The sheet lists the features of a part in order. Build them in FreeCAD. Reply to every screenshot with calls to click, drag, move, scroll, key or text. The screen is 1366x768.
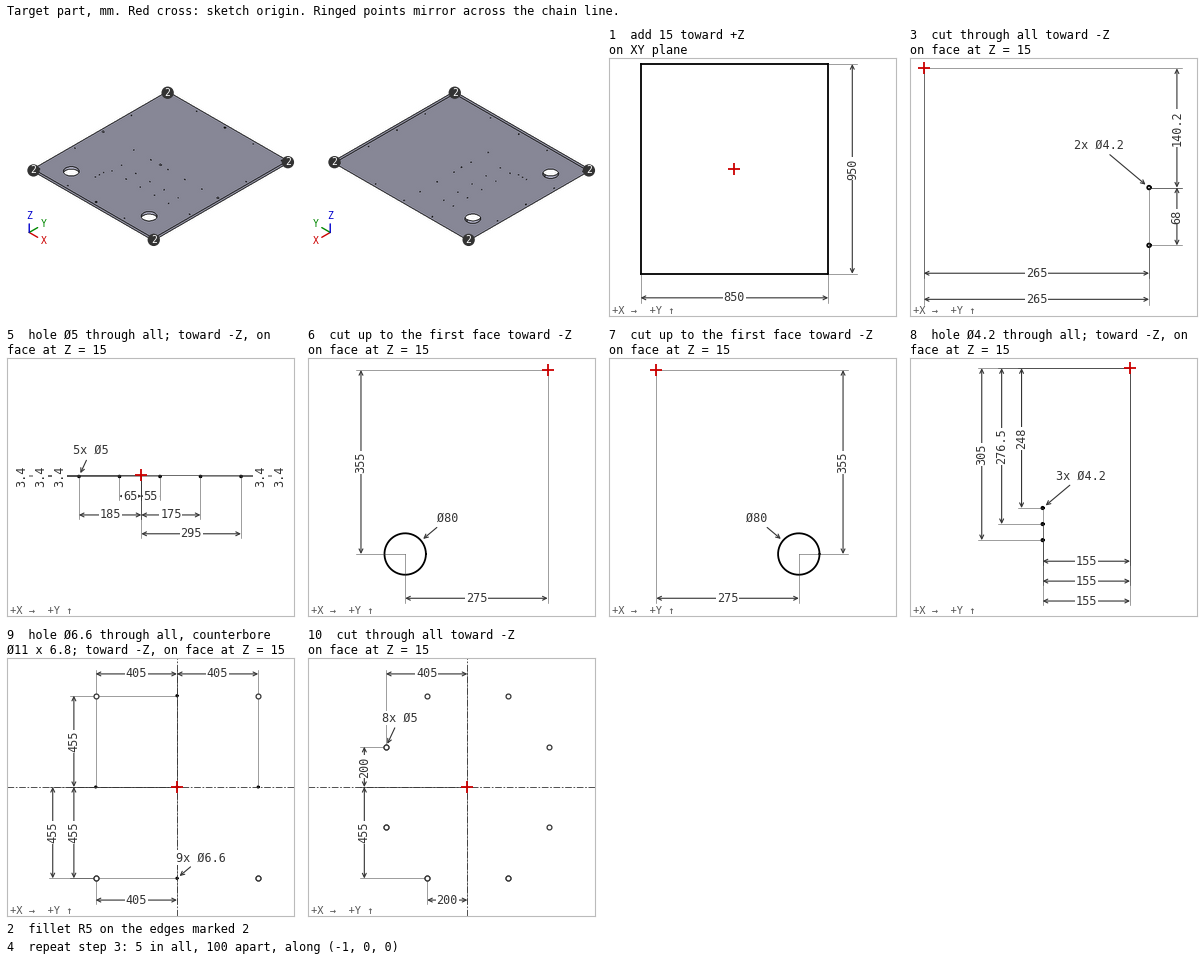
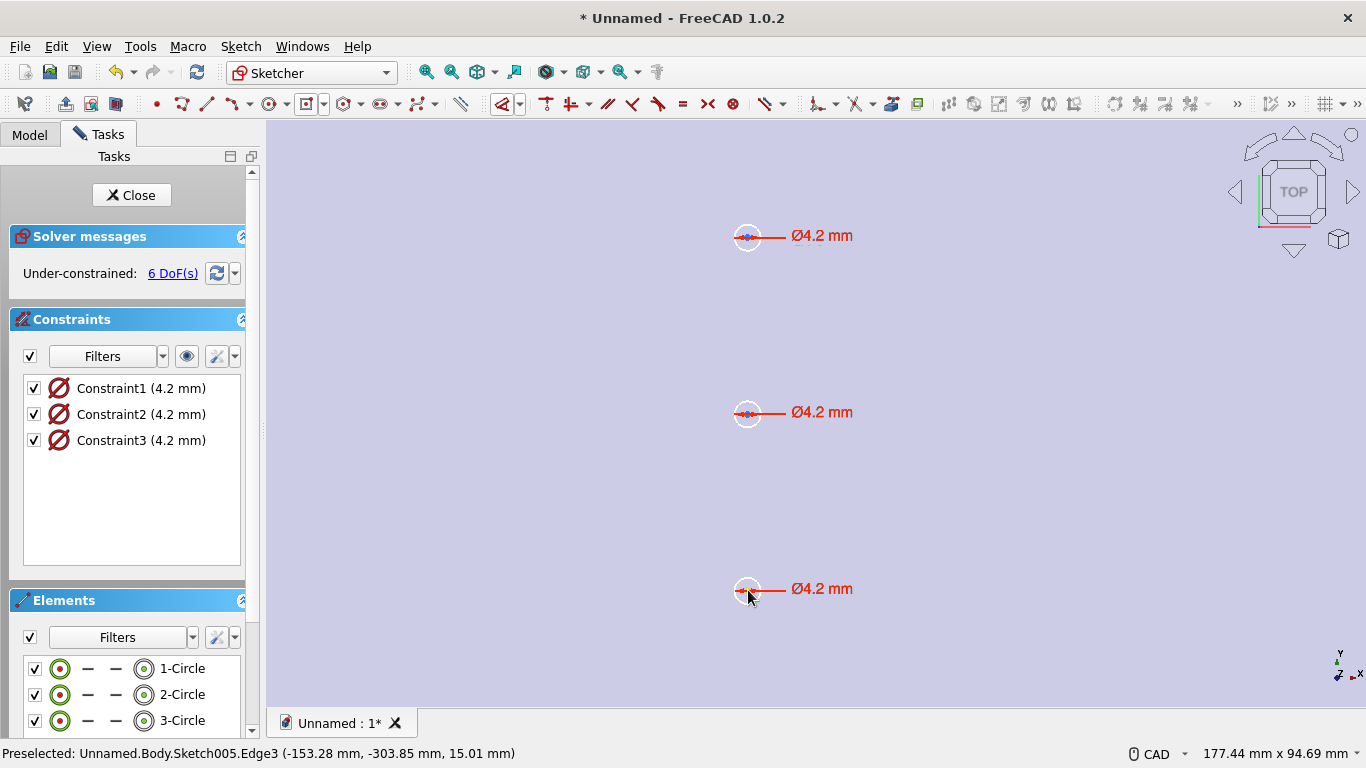
click(748, 238)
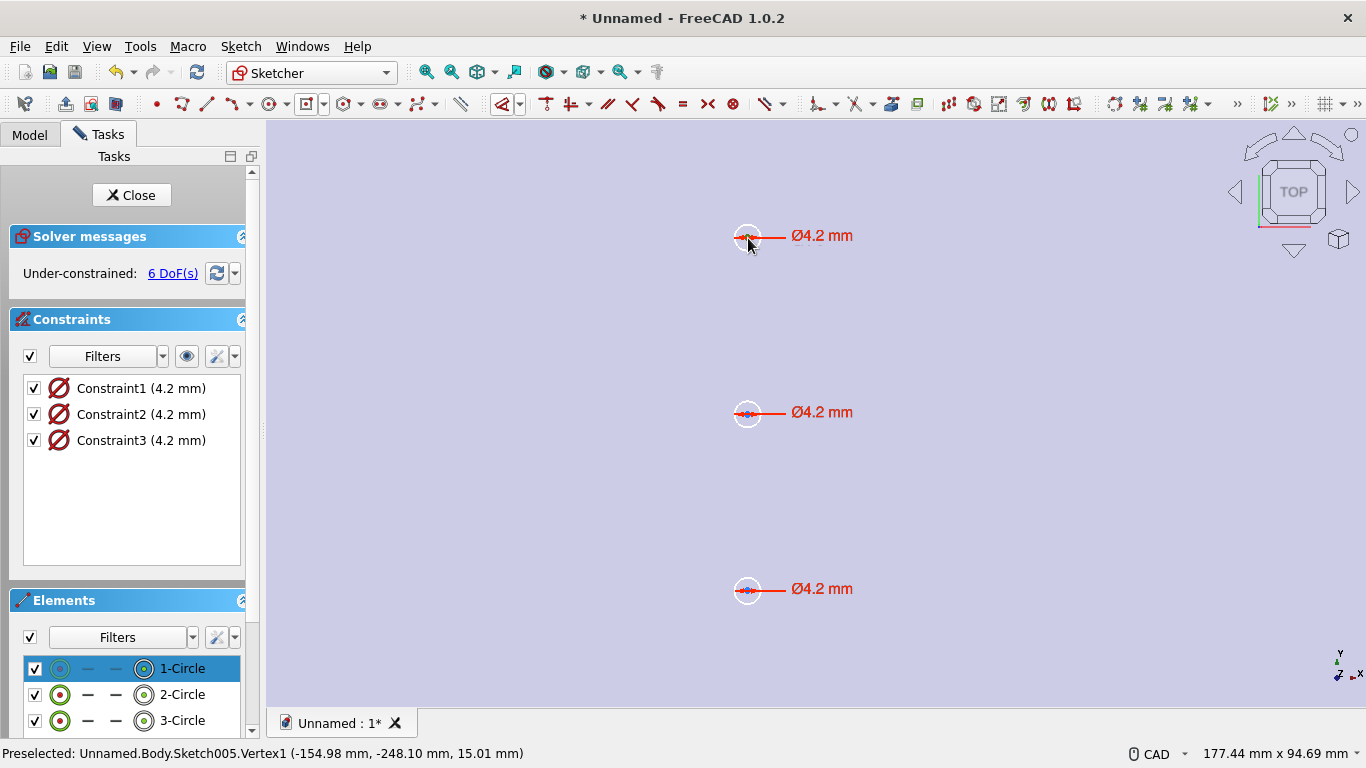
click(520, 104)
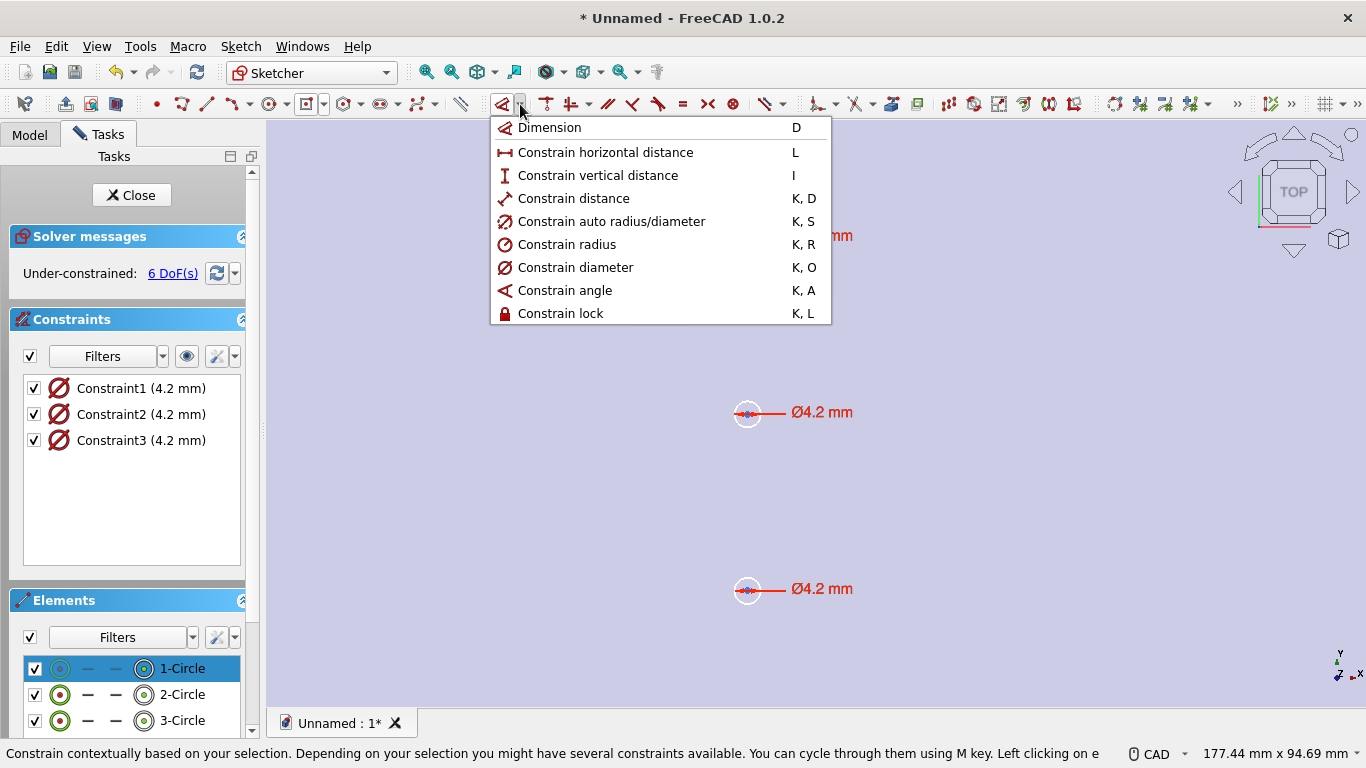
click(661, 152)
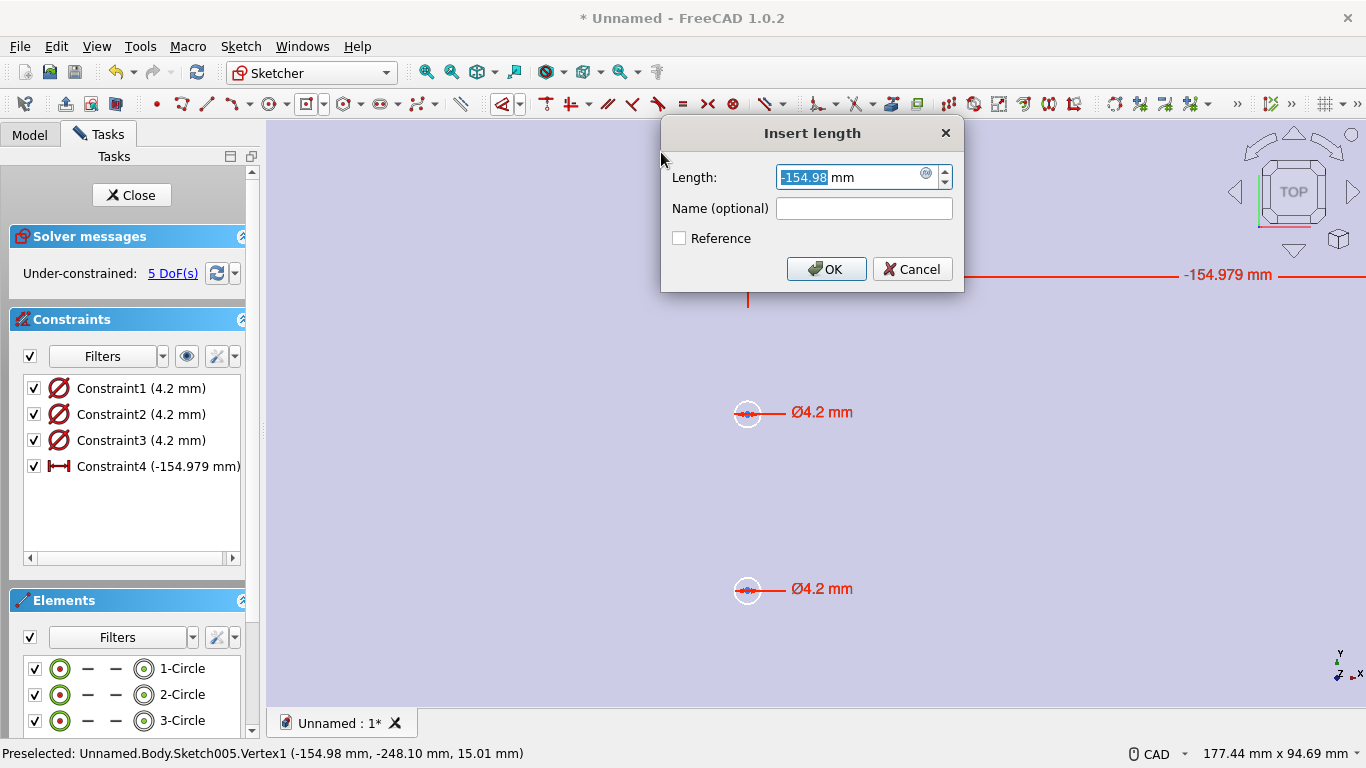
text(-155)
key(Return)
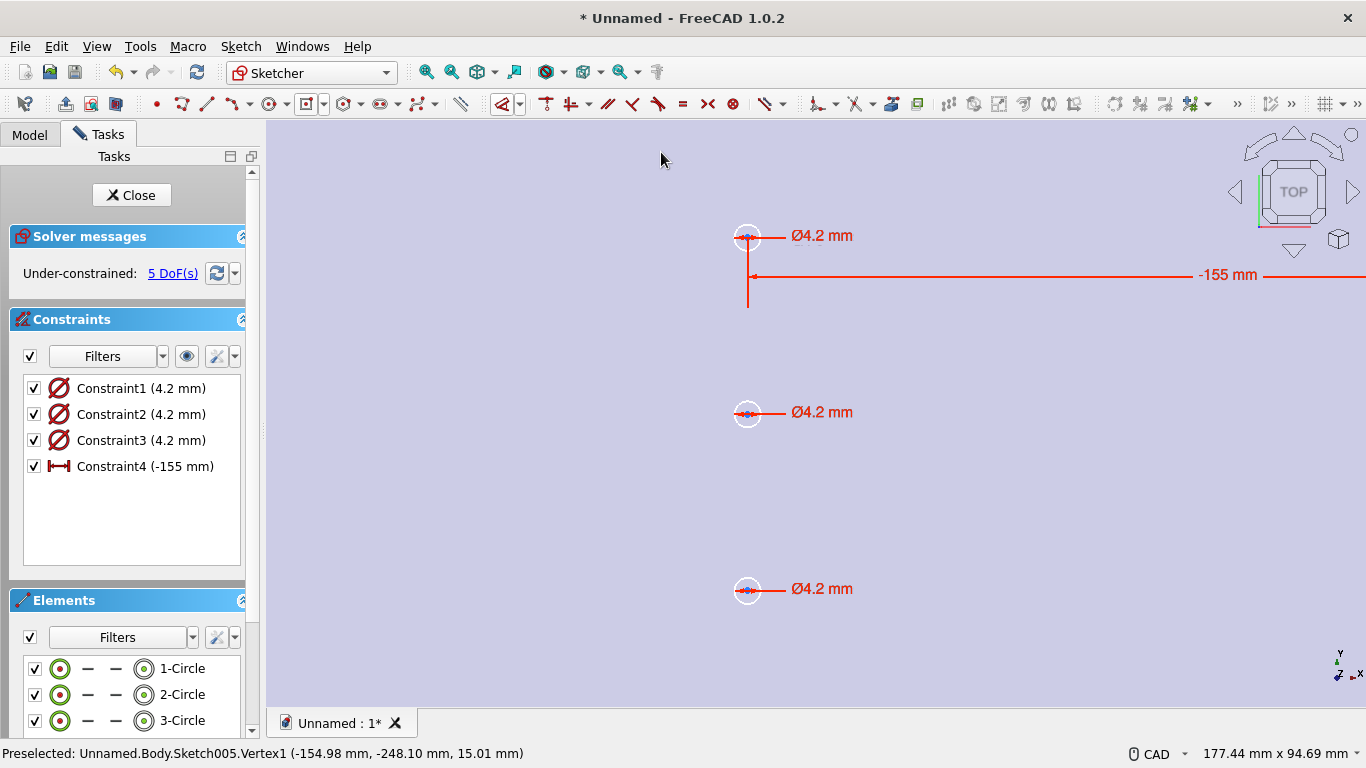
click(748, 238)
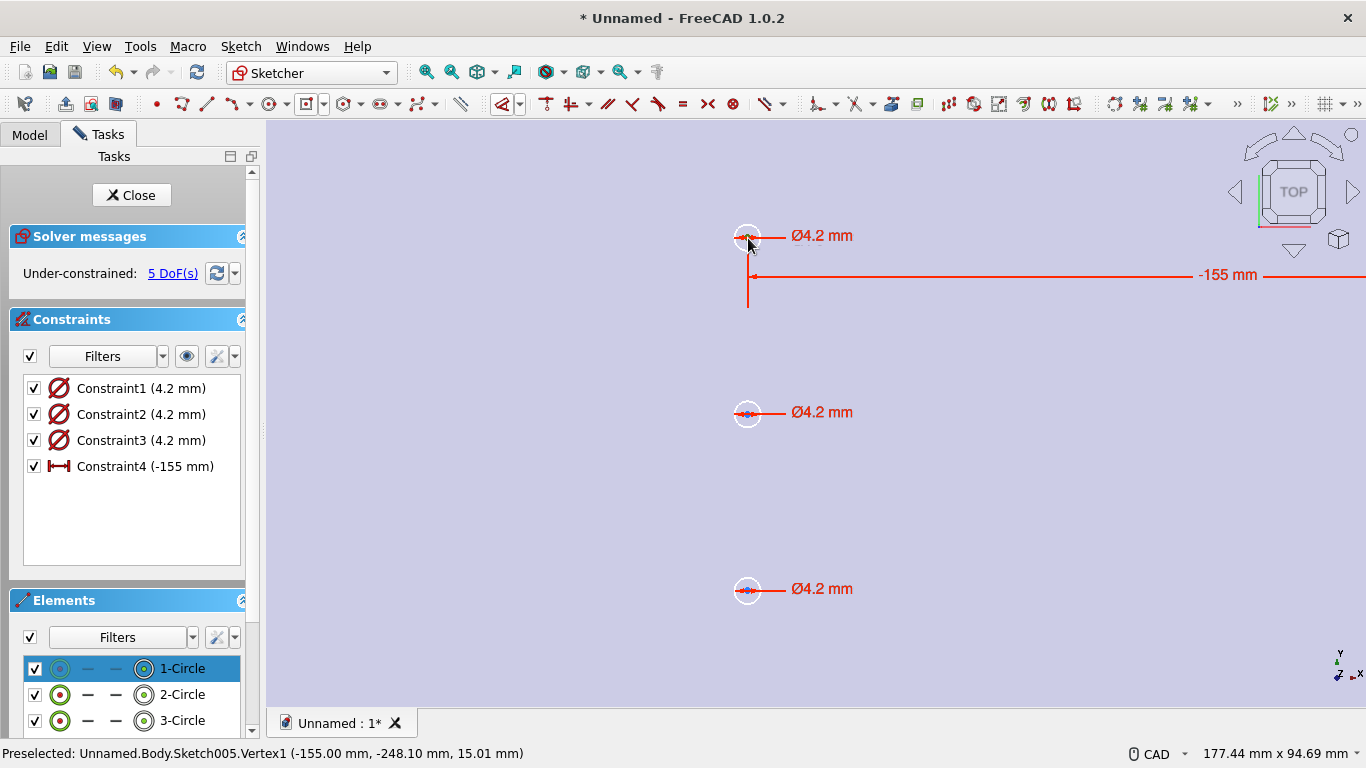
key(i)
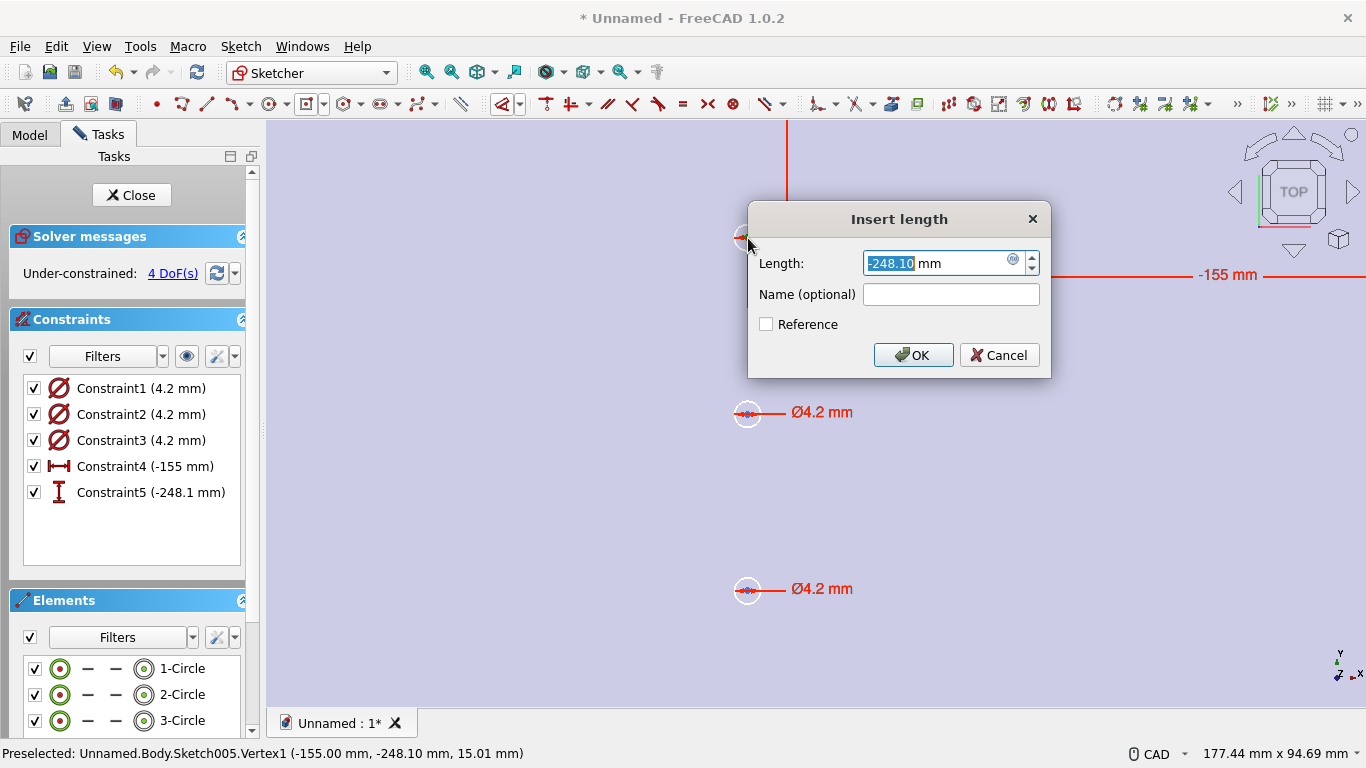
text(-248)
key(Return)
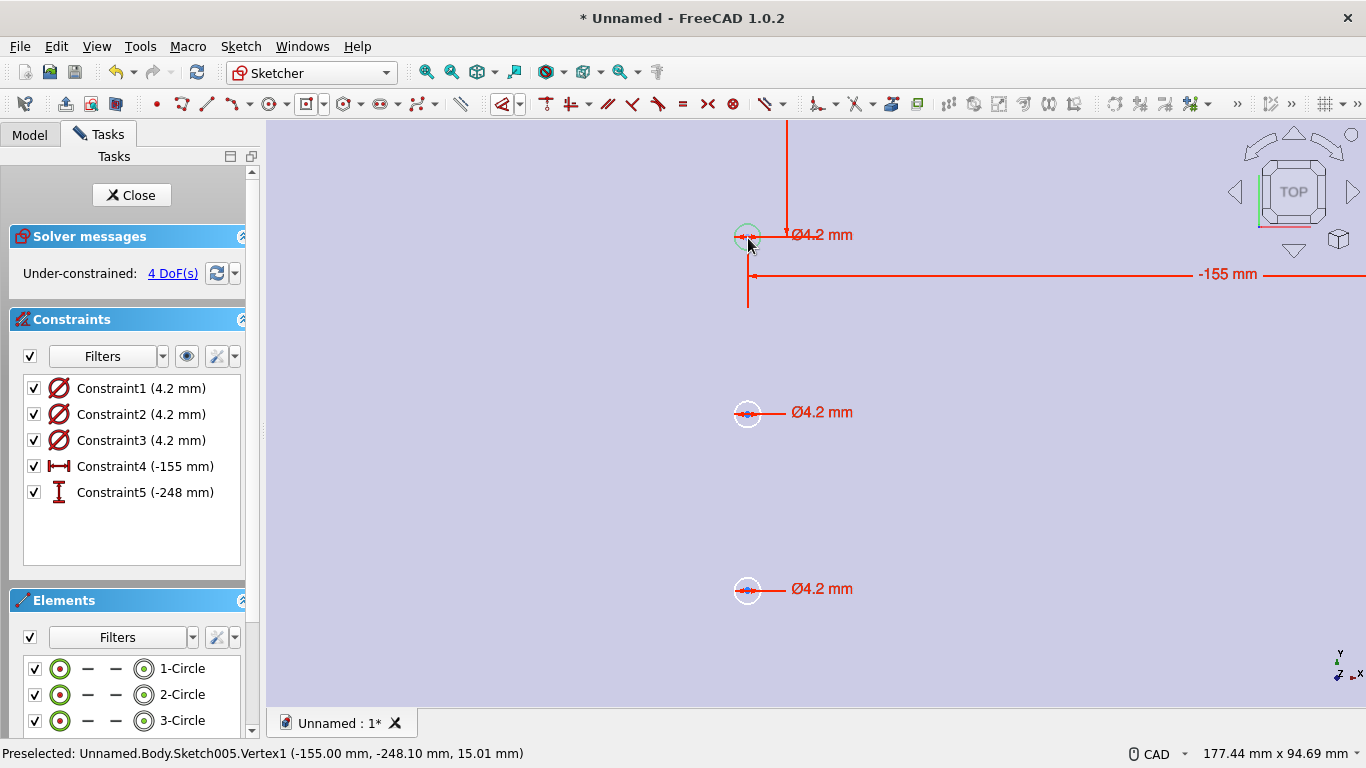
click(748, 414)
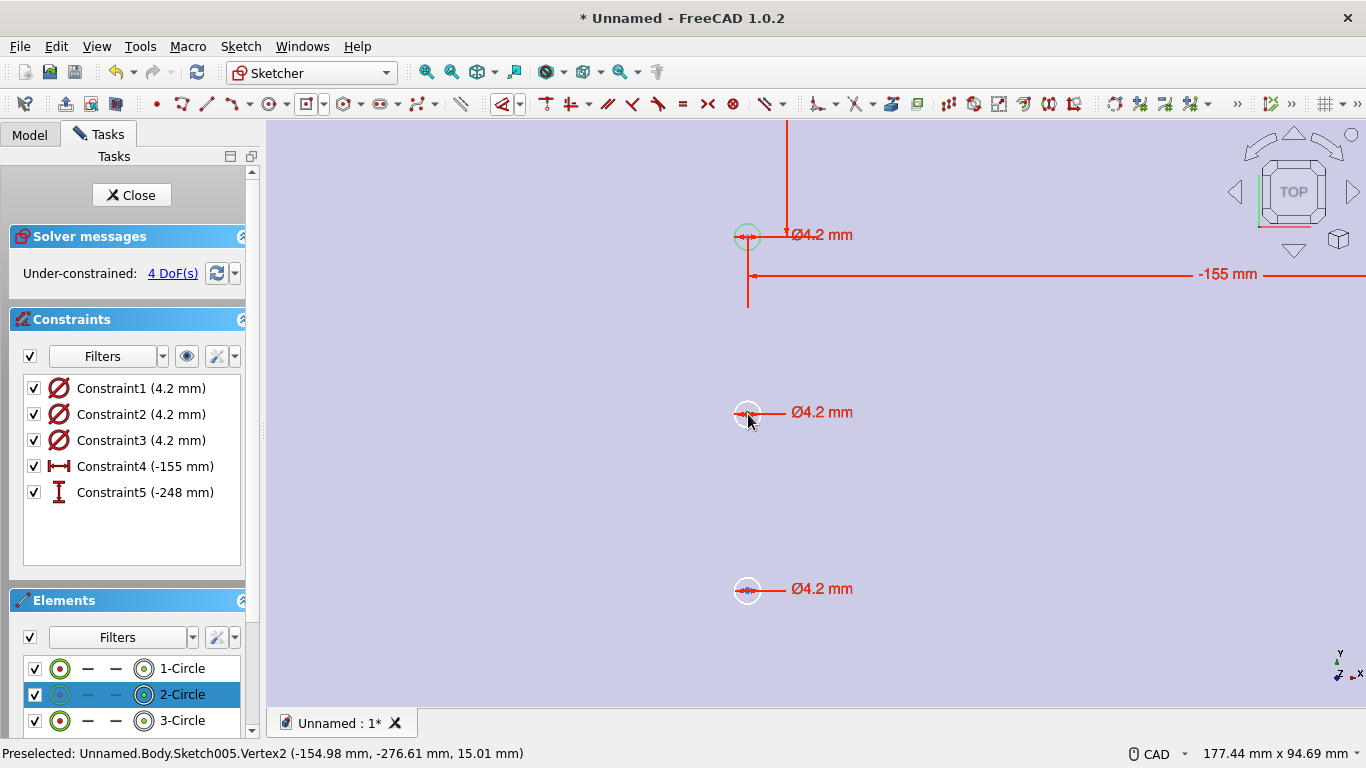
click(520, 104)